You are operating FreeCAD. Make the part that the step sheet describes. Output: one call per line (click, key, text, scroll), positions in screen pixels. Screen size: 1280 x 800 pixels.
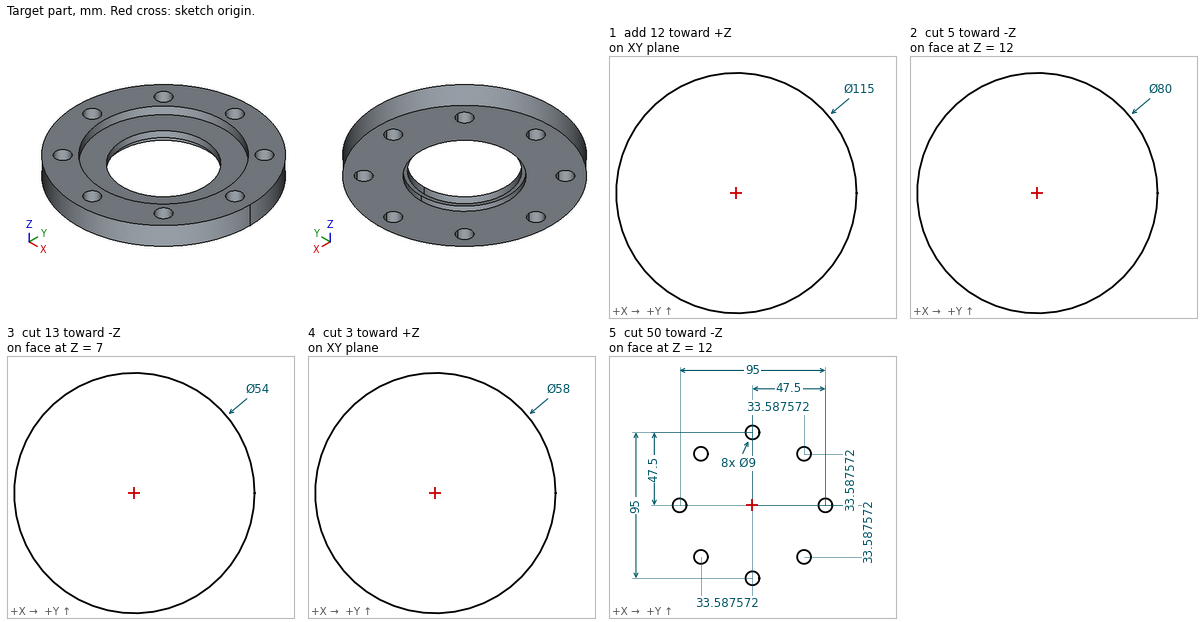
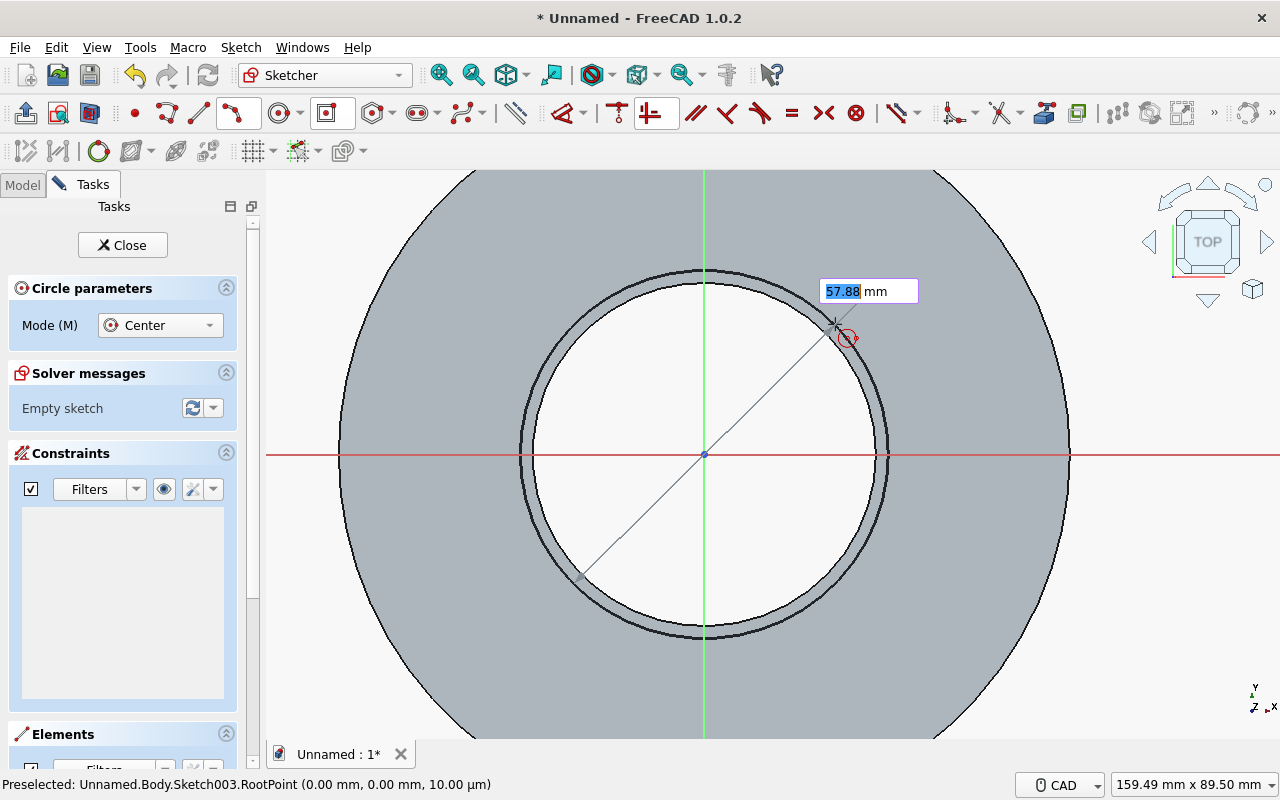
text(58)
key(Return)
key(Escape)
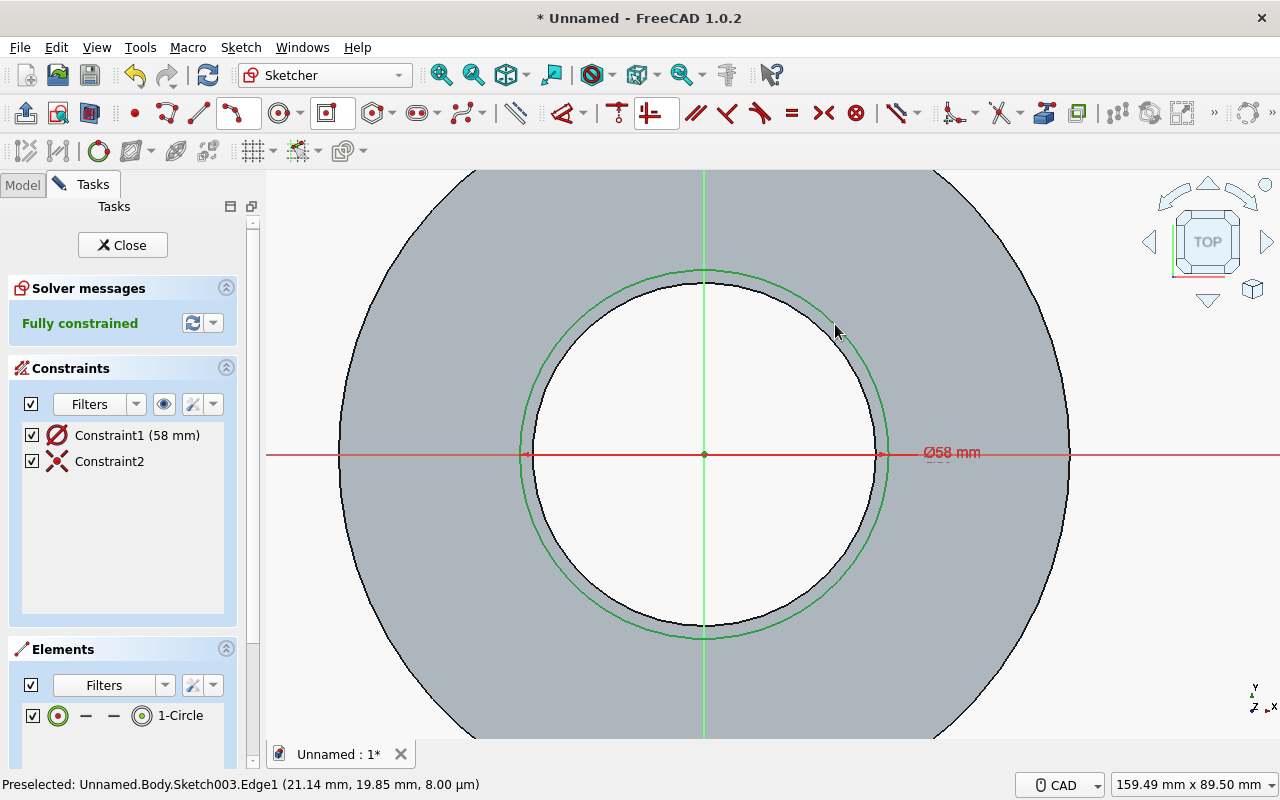
click(123, 245)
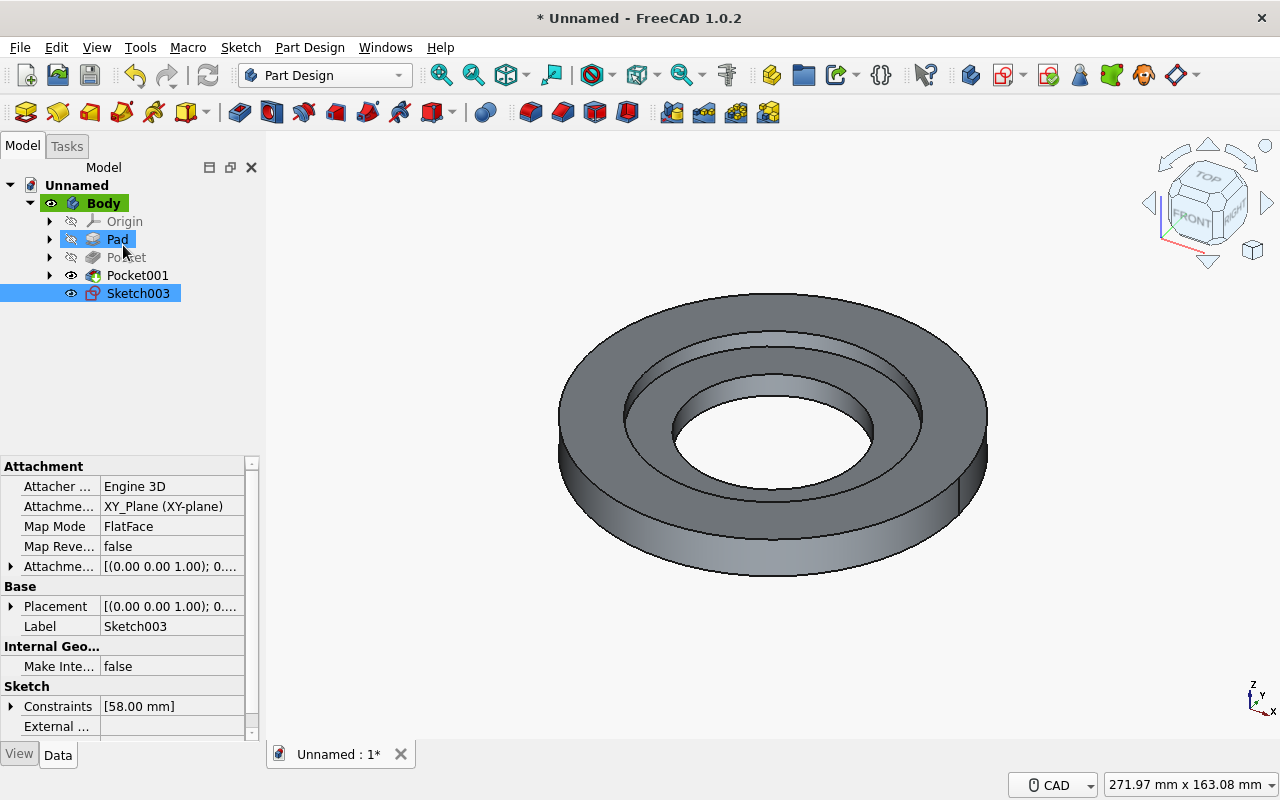
click(240, 112)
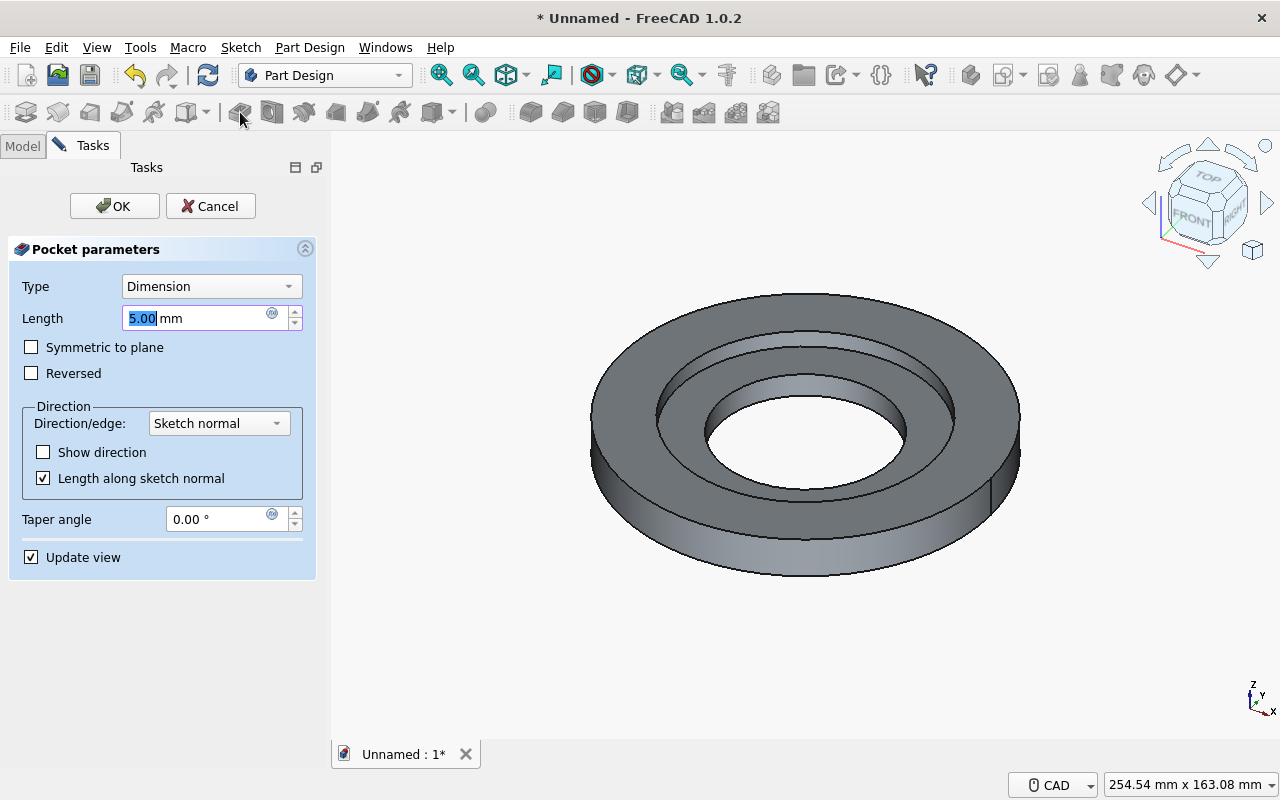
text(3)
key(Tab)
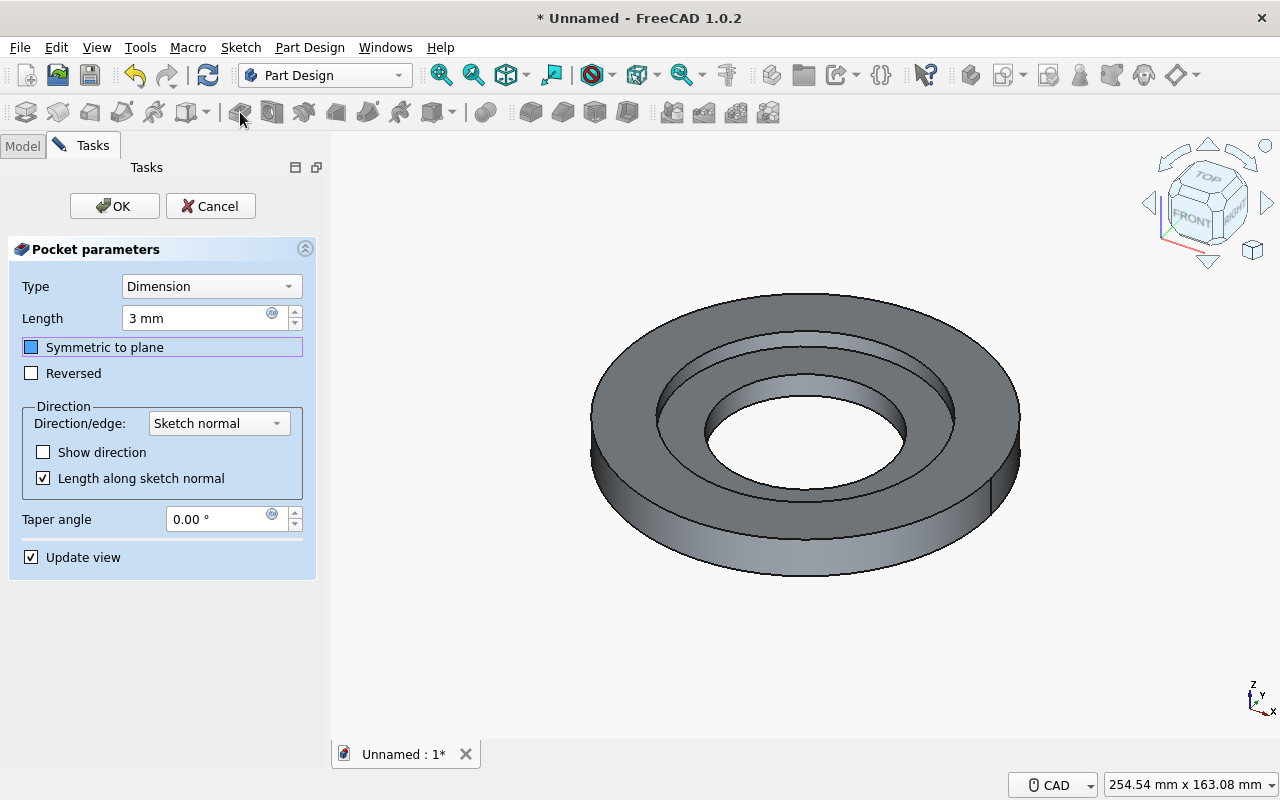
click(30, 373)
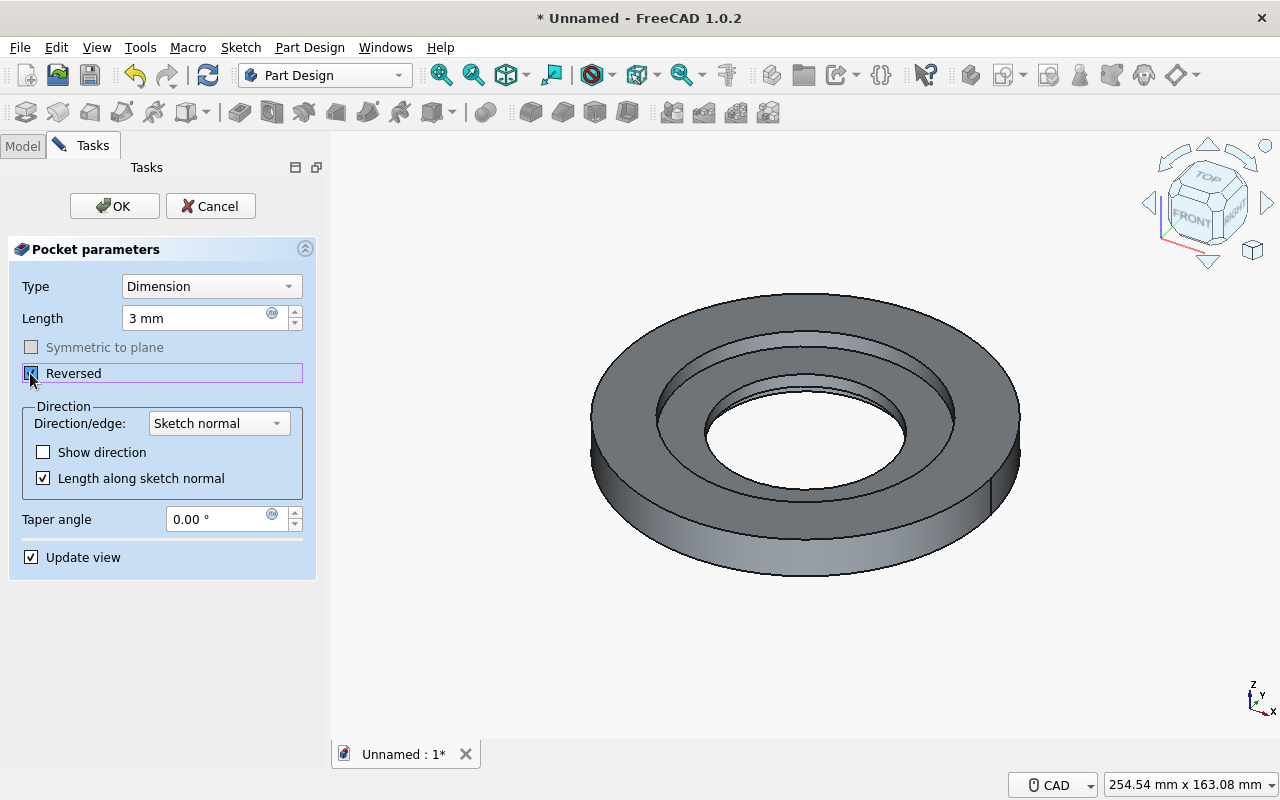
click(115, 206)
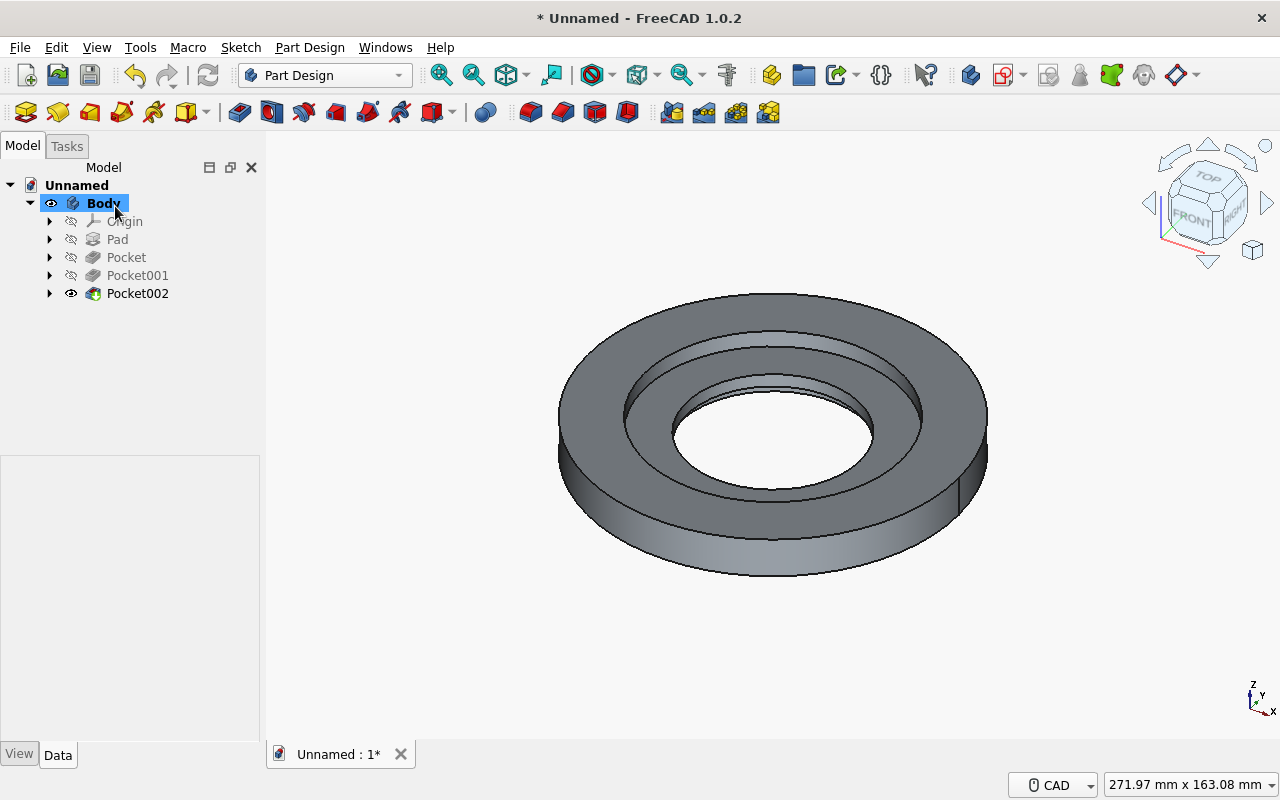
click(681, 507)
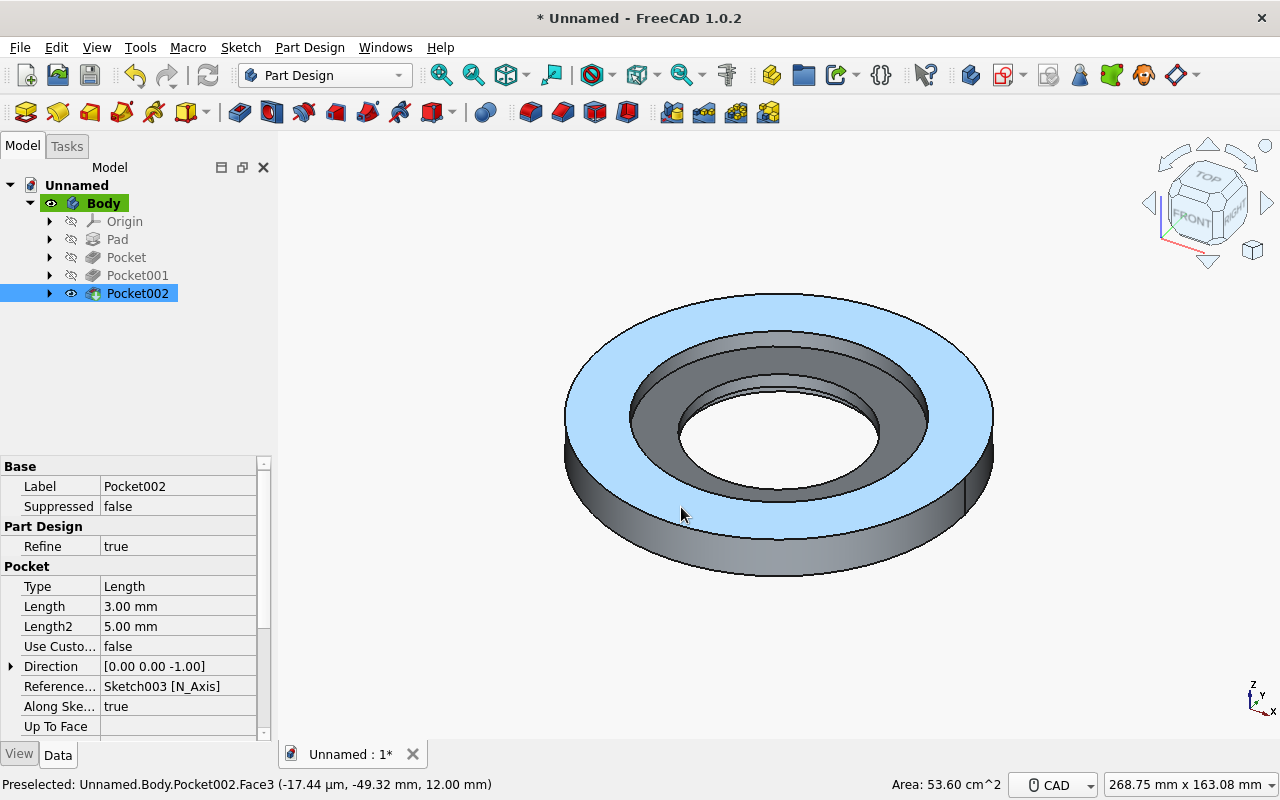
click(1004, 76)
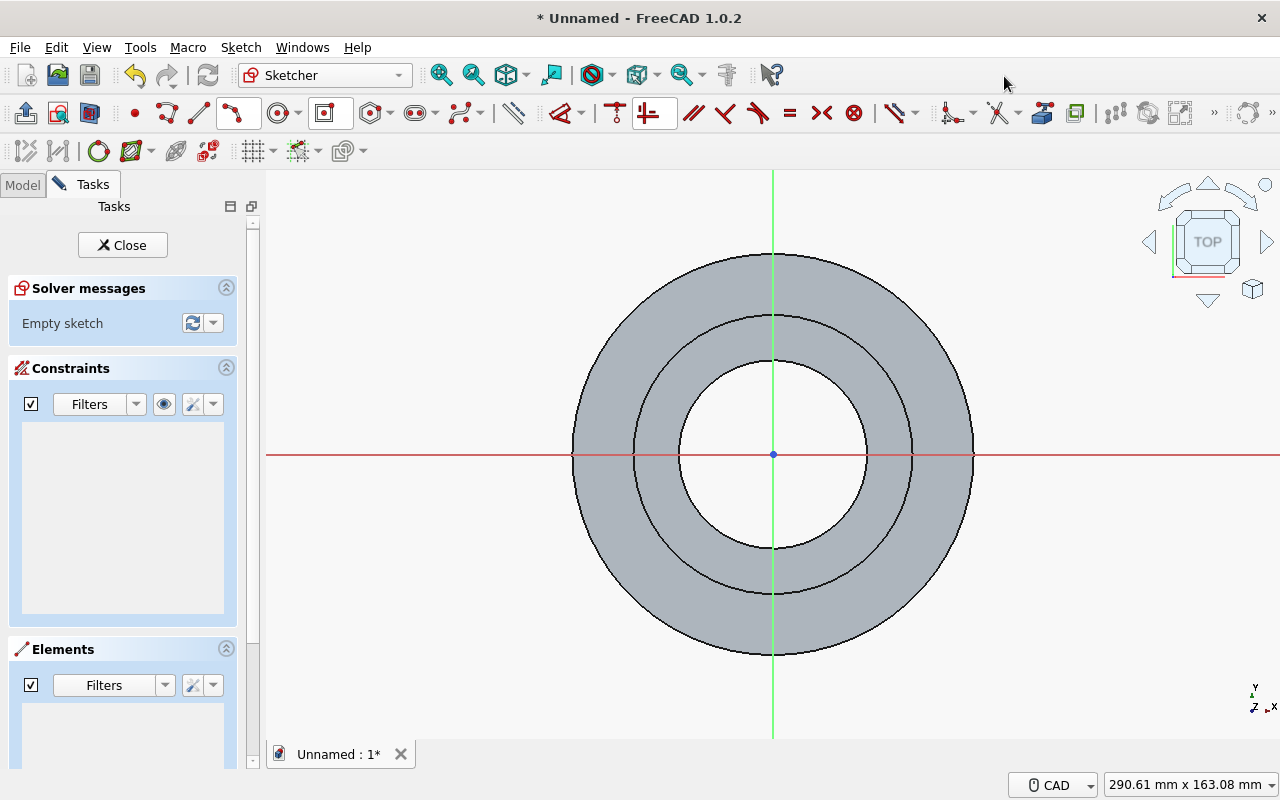
click(278, 114)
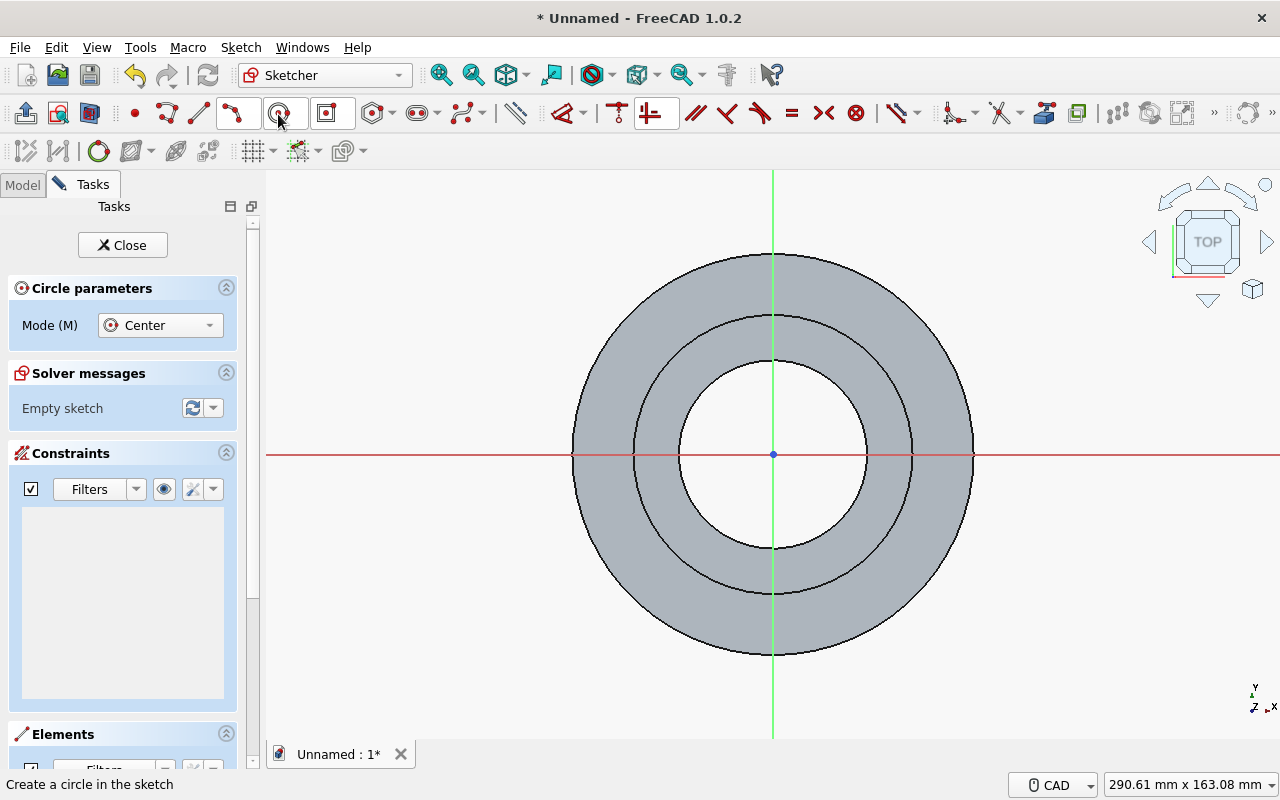
scroll(773, 289, up, 2)